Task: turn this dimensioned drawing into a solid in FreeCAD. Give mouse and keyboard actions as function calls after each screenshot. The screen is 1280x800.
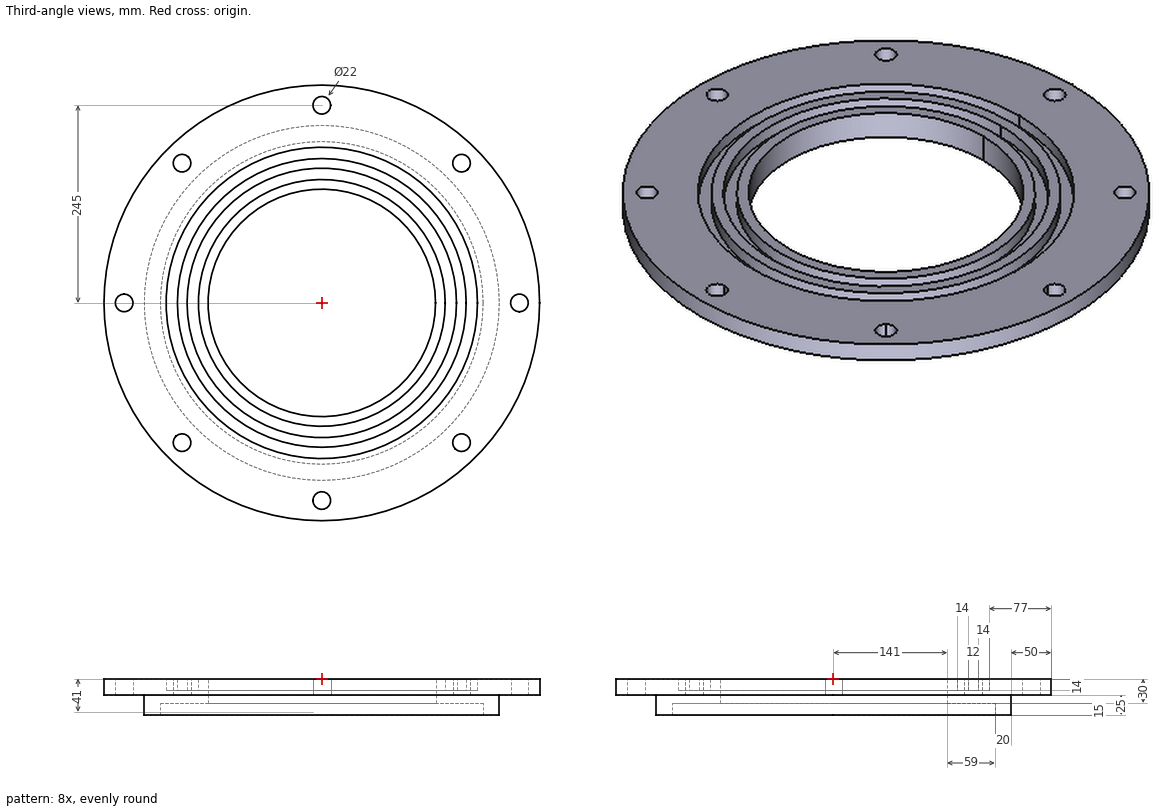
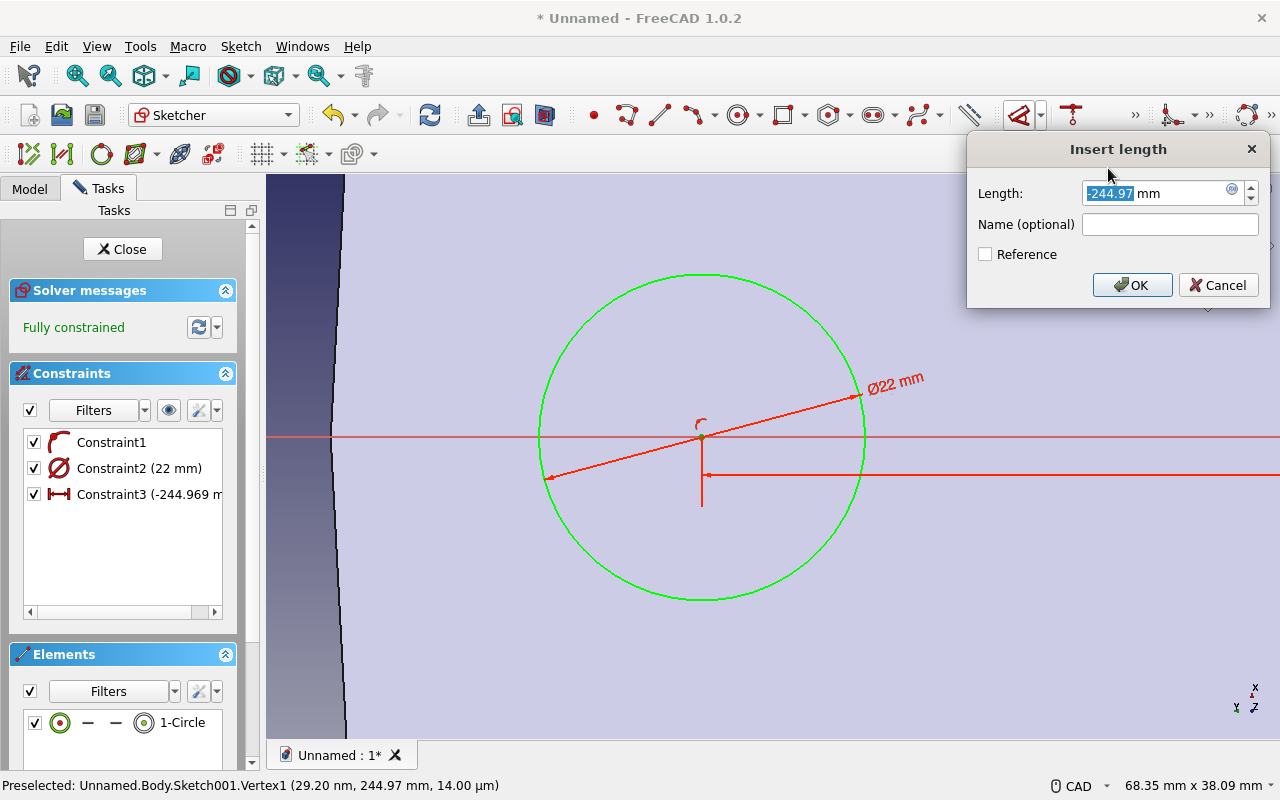
text(-245)
key(Return)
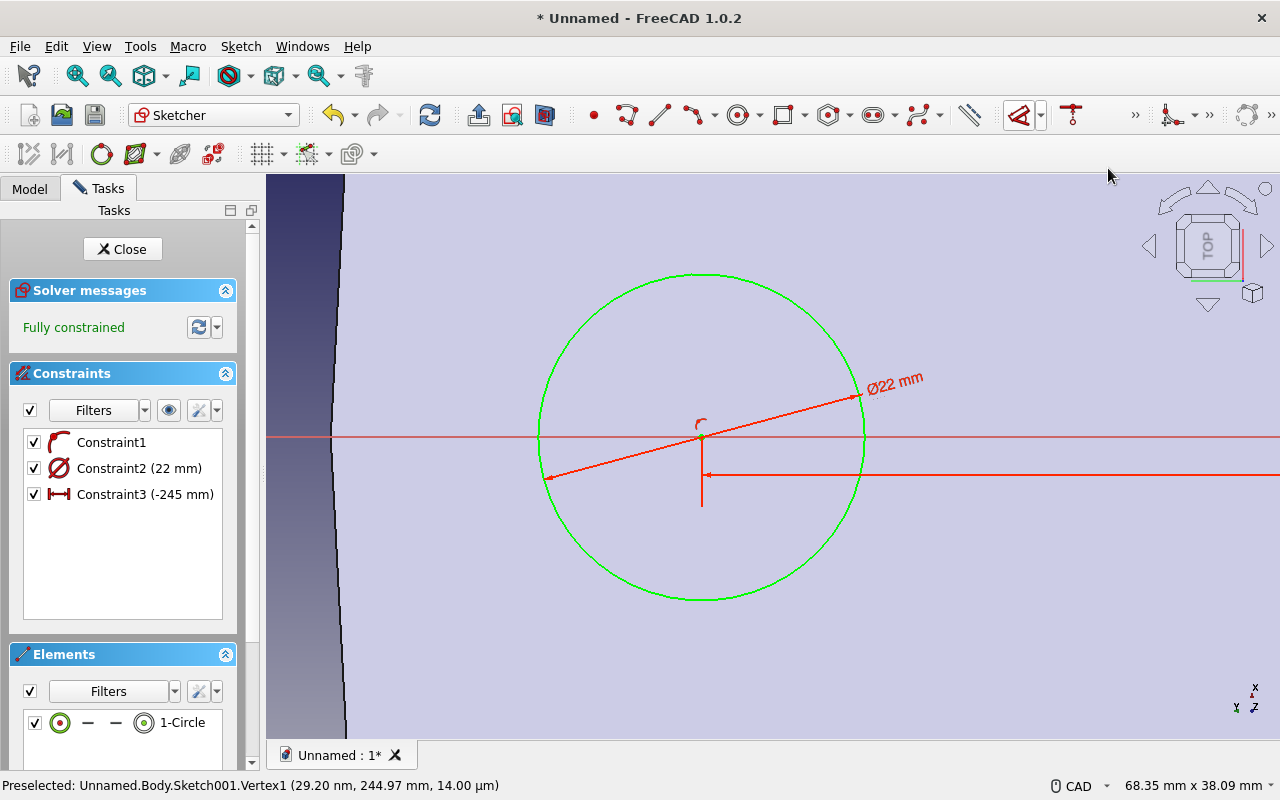
click(123, 249)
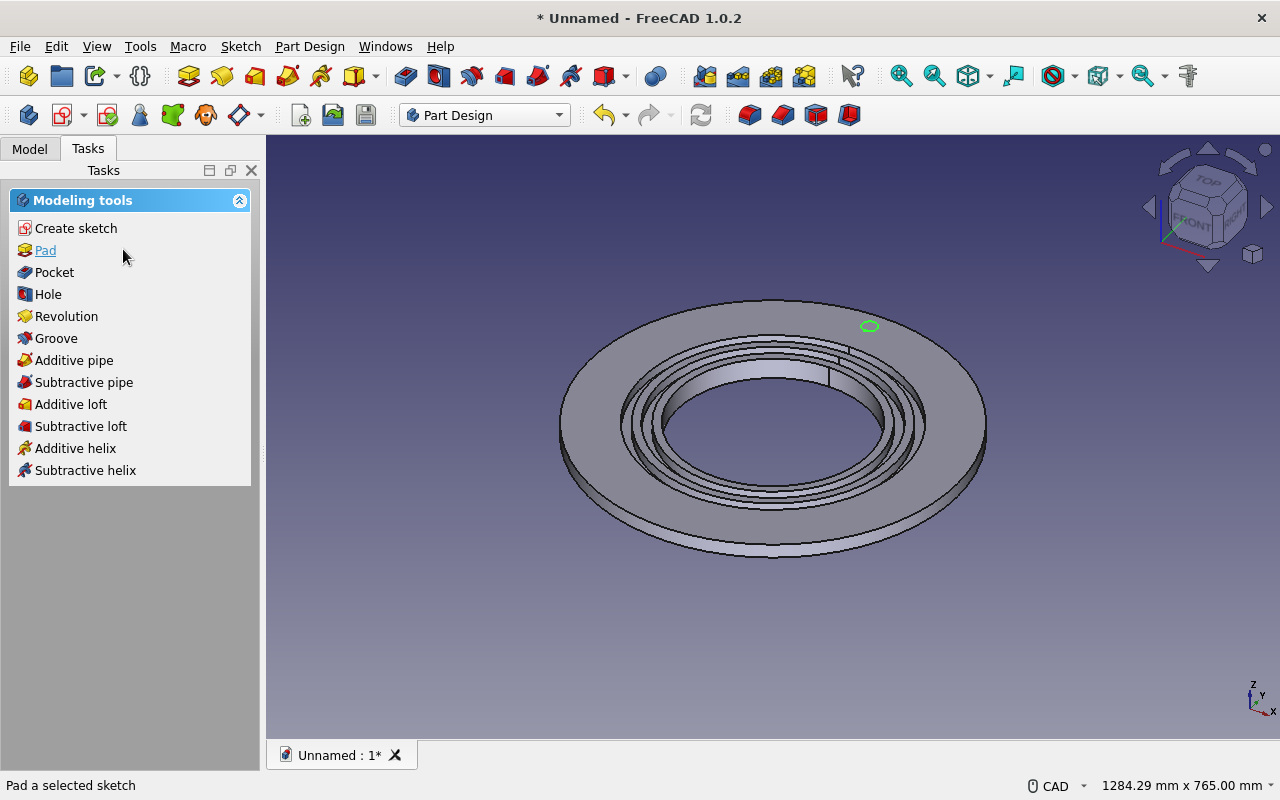
click(406, 76)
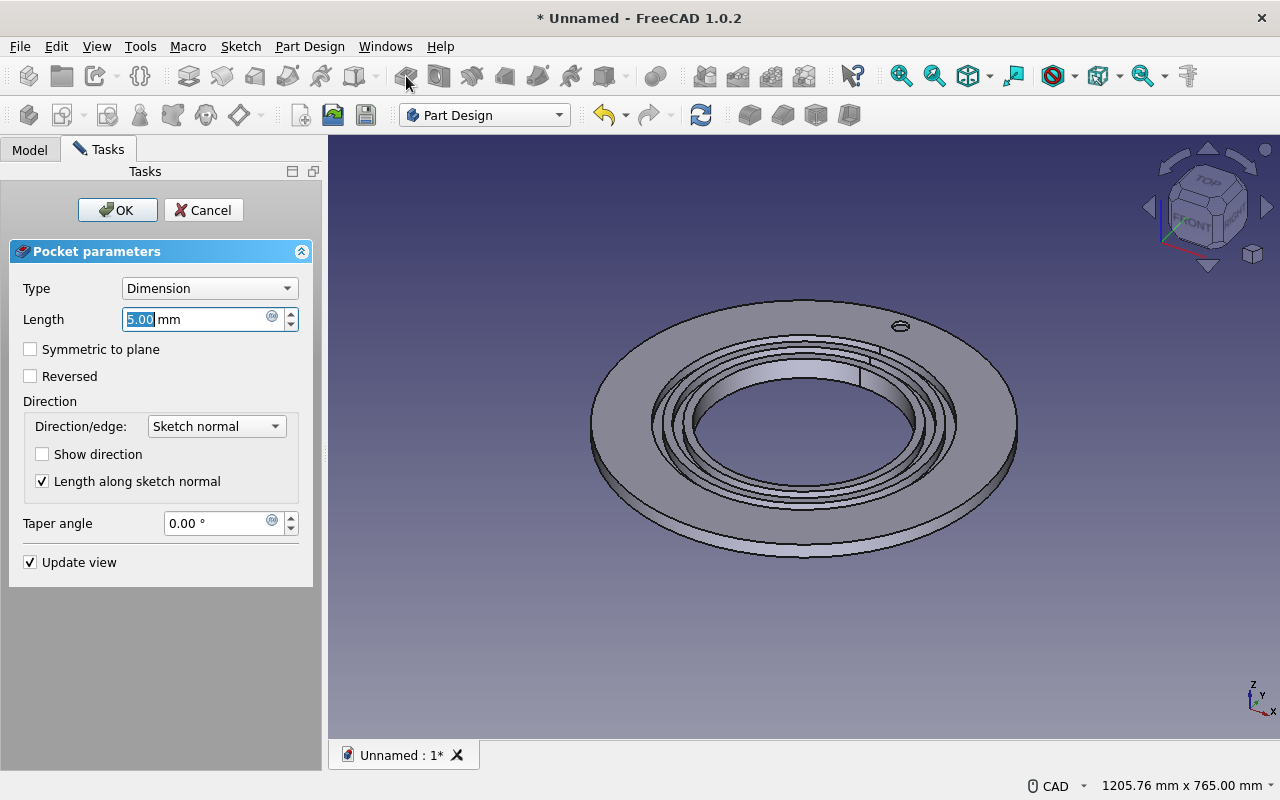
text(41)
key(Tab)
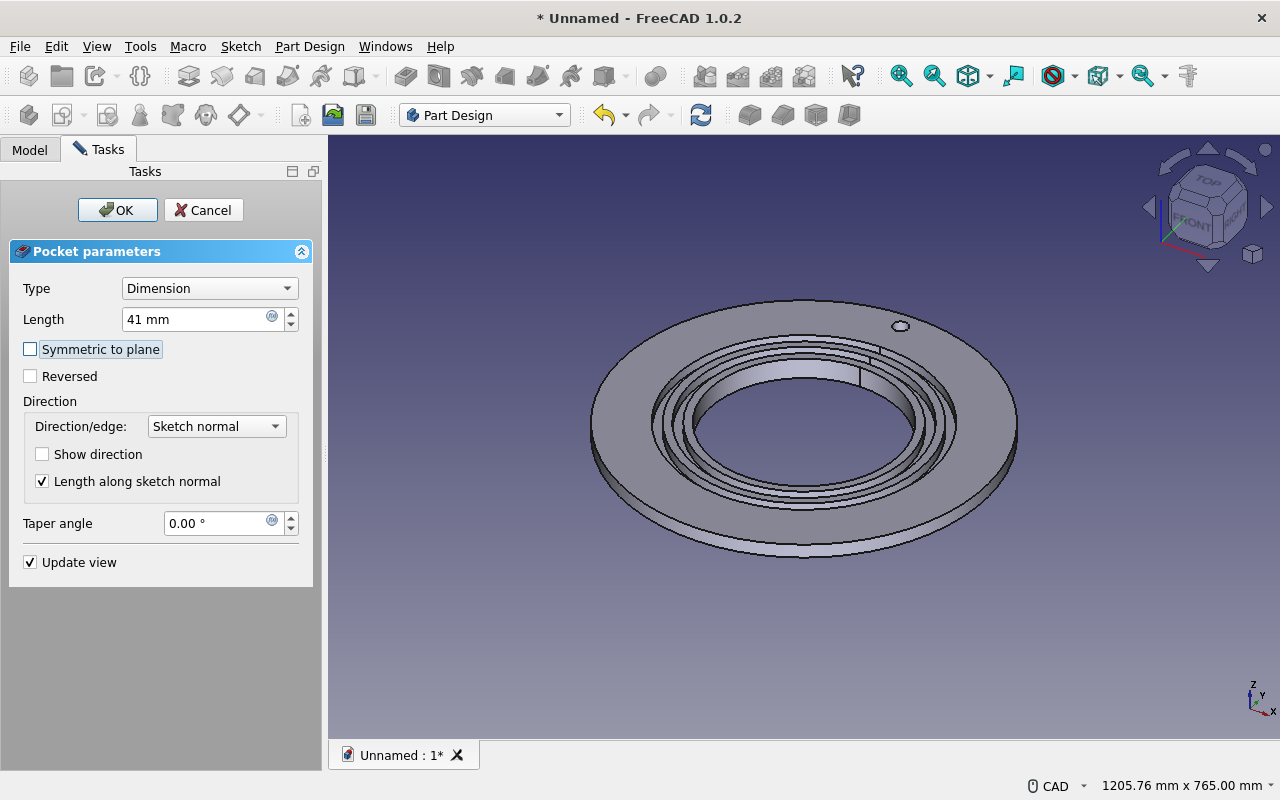
click(118, 210)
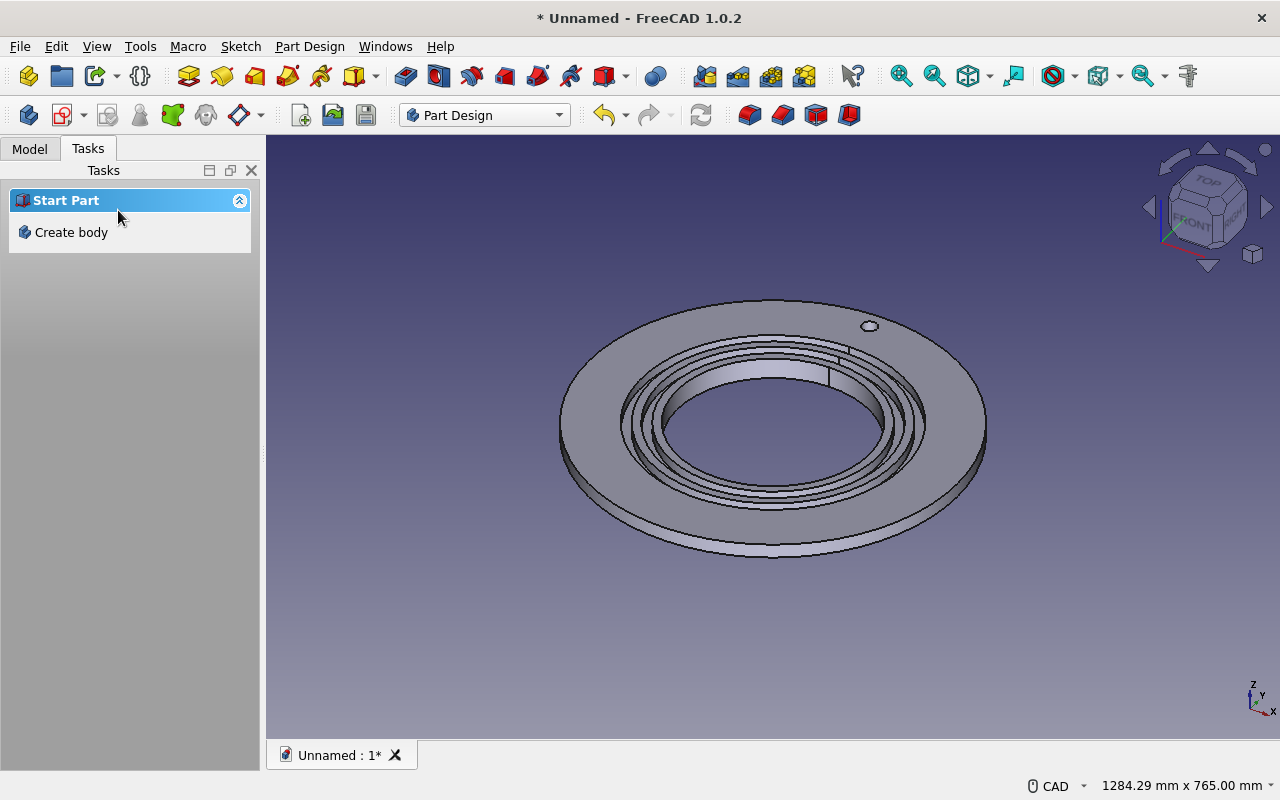
click(30, 148)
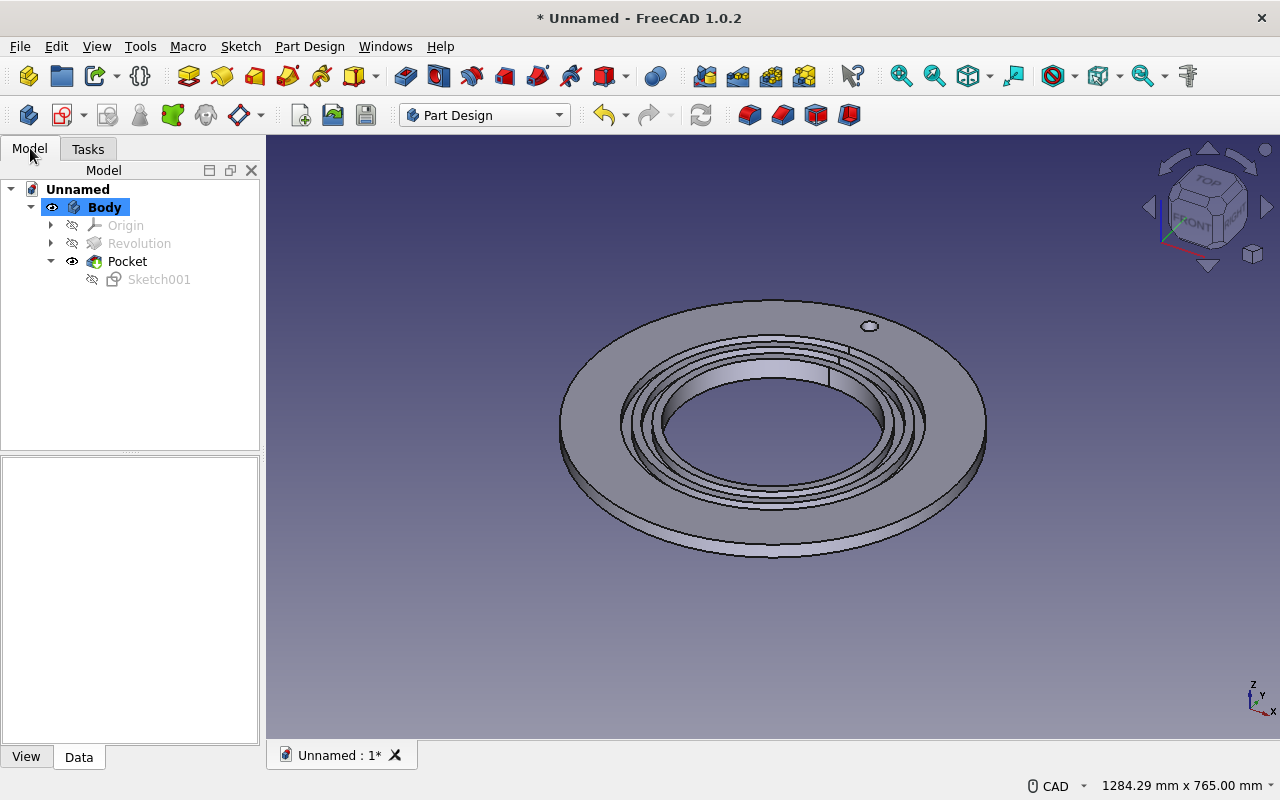
click(117, 261)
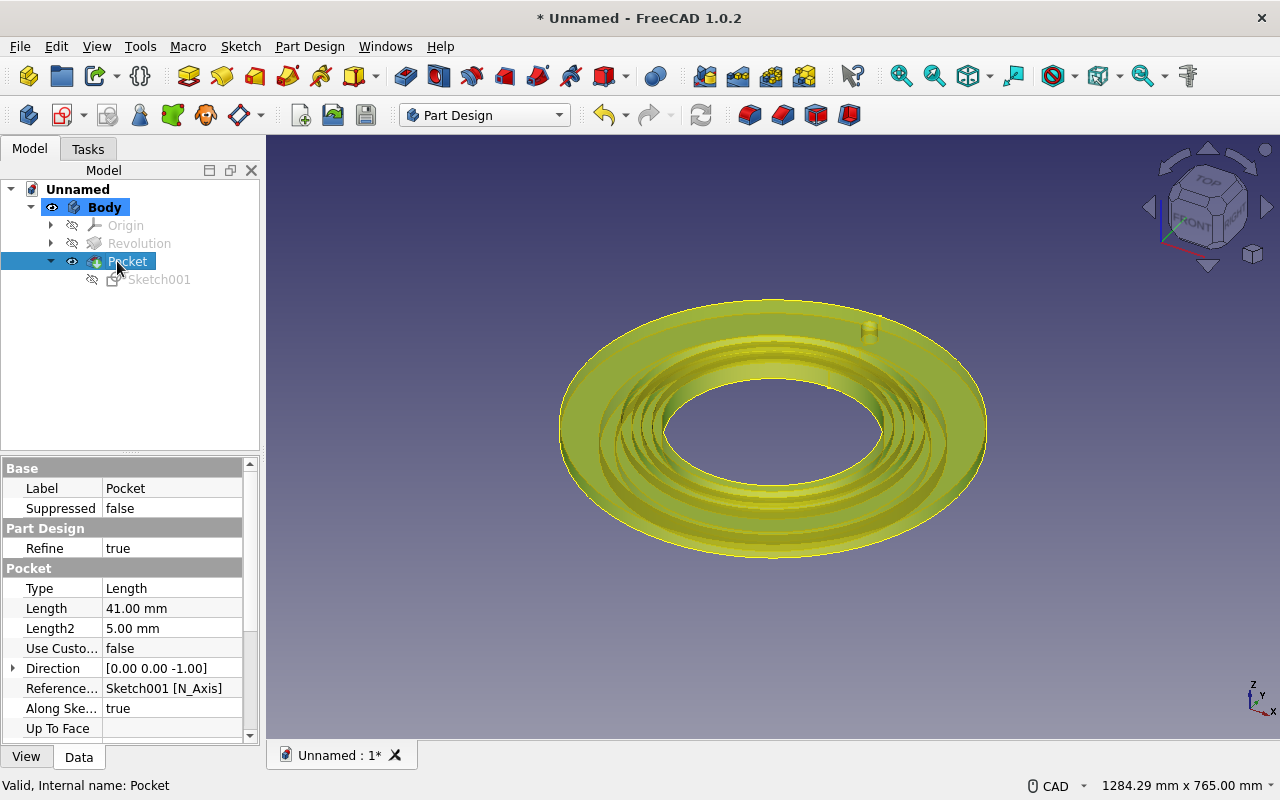
click(771, 76)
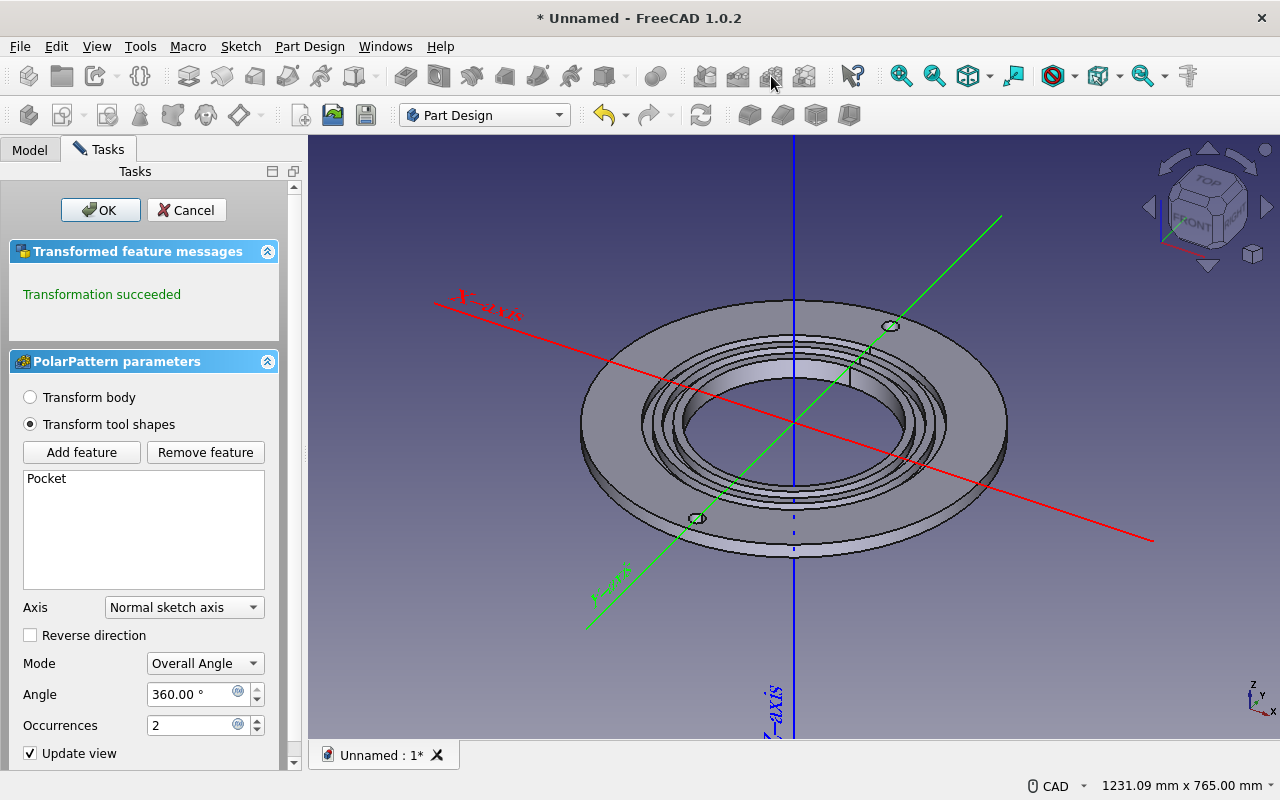
click(185, 608)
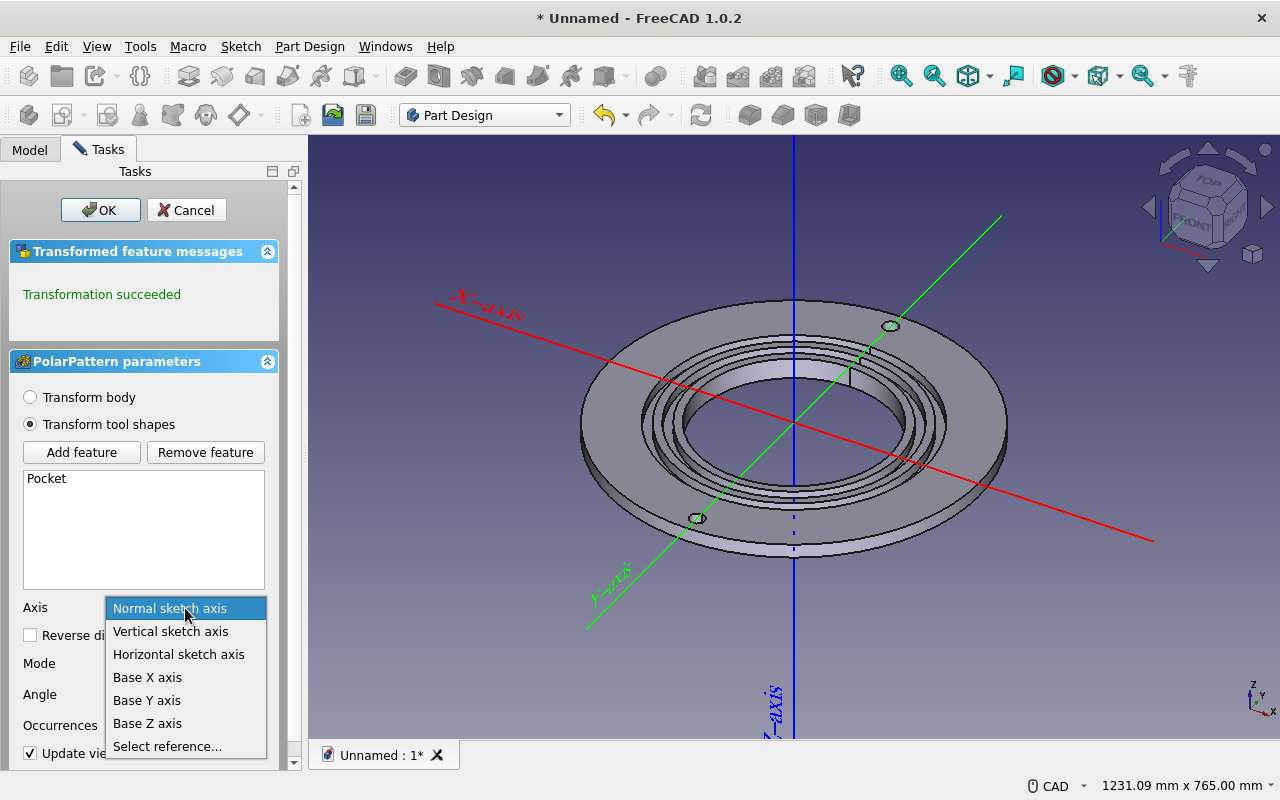
click(184, 724)